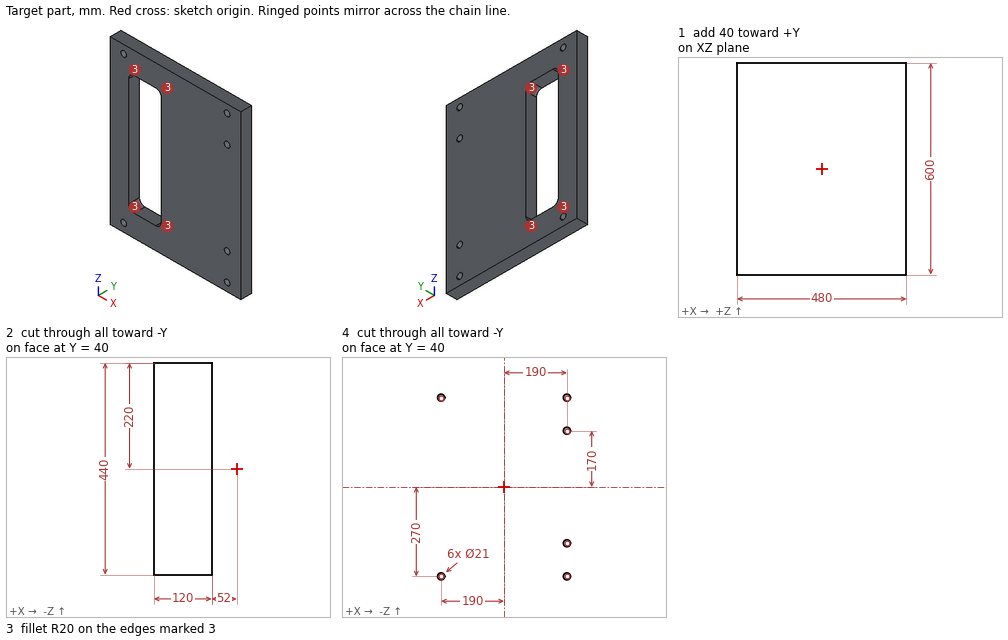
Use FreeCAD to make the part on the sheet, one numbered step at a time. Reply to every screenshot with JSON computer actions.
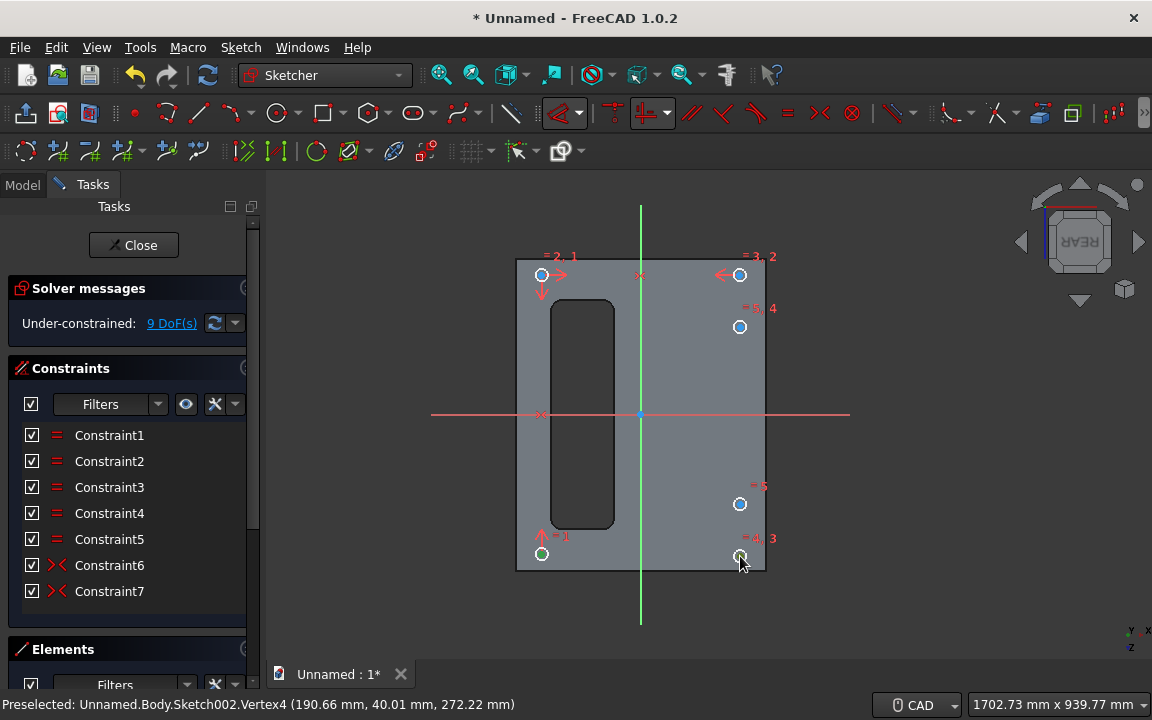
{"action": "left_click", "coordinate": [641, 600]}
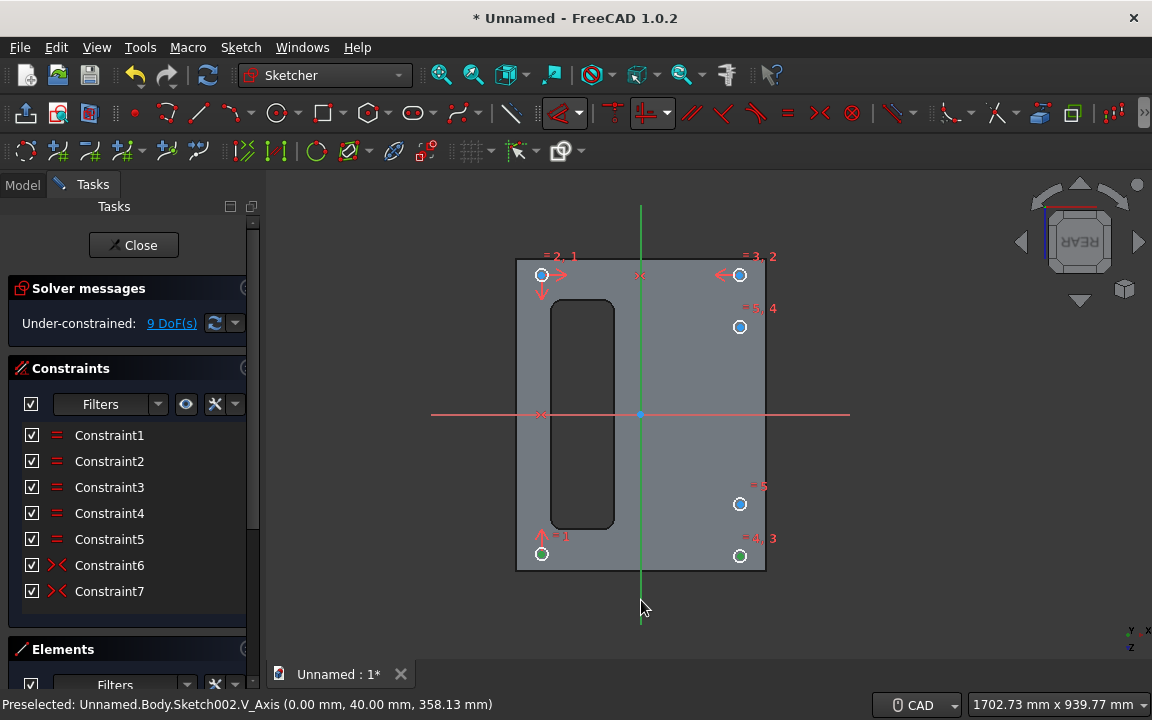
{"action": "left_click", "coordinate": [820, 114]}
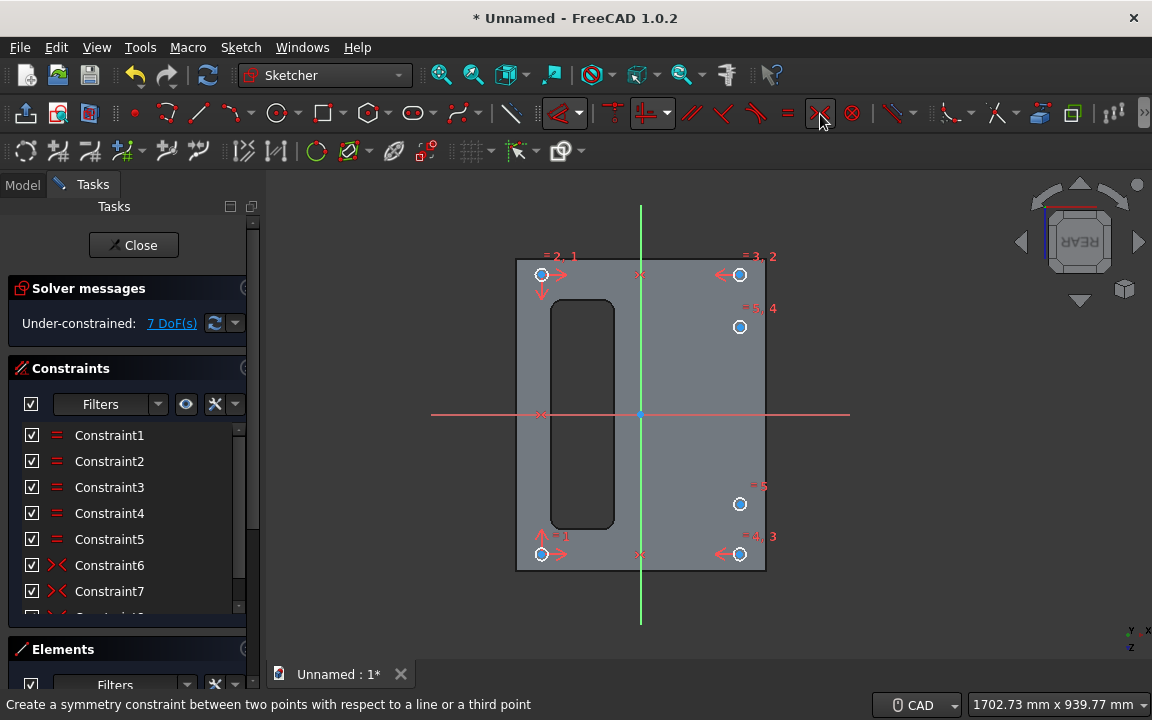
{"action": "left_click", "coordinate": [740, 327]}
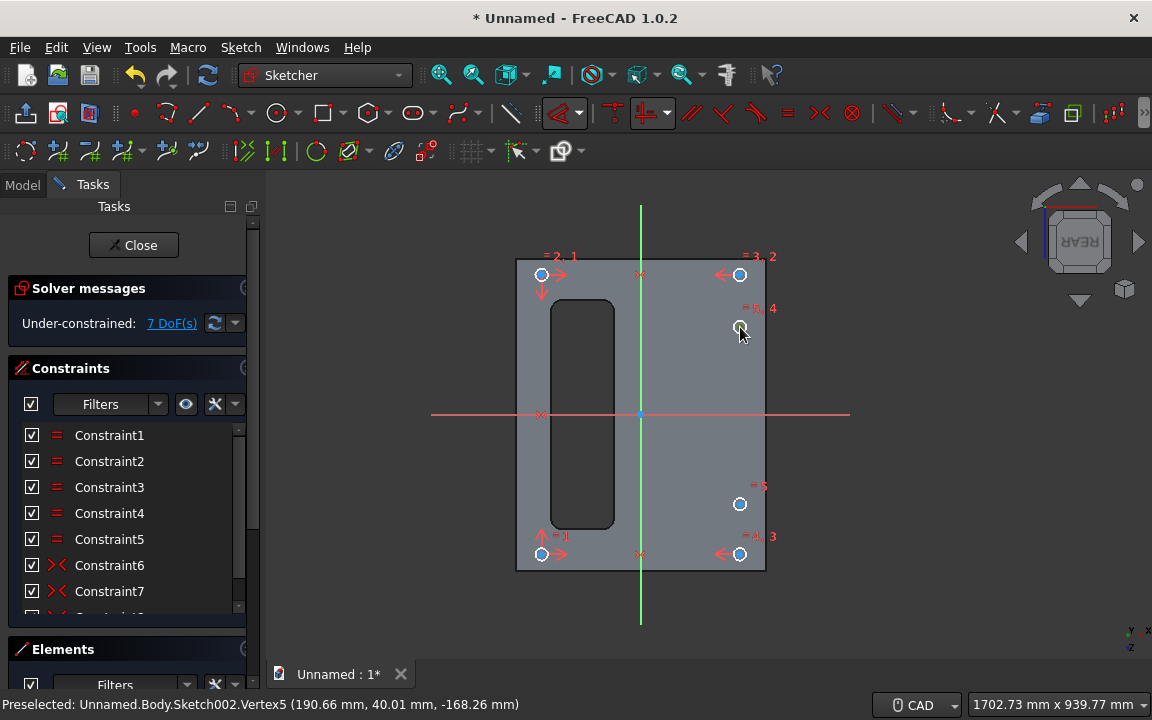
{"action": "left_click", "coordinate": [740, 504]}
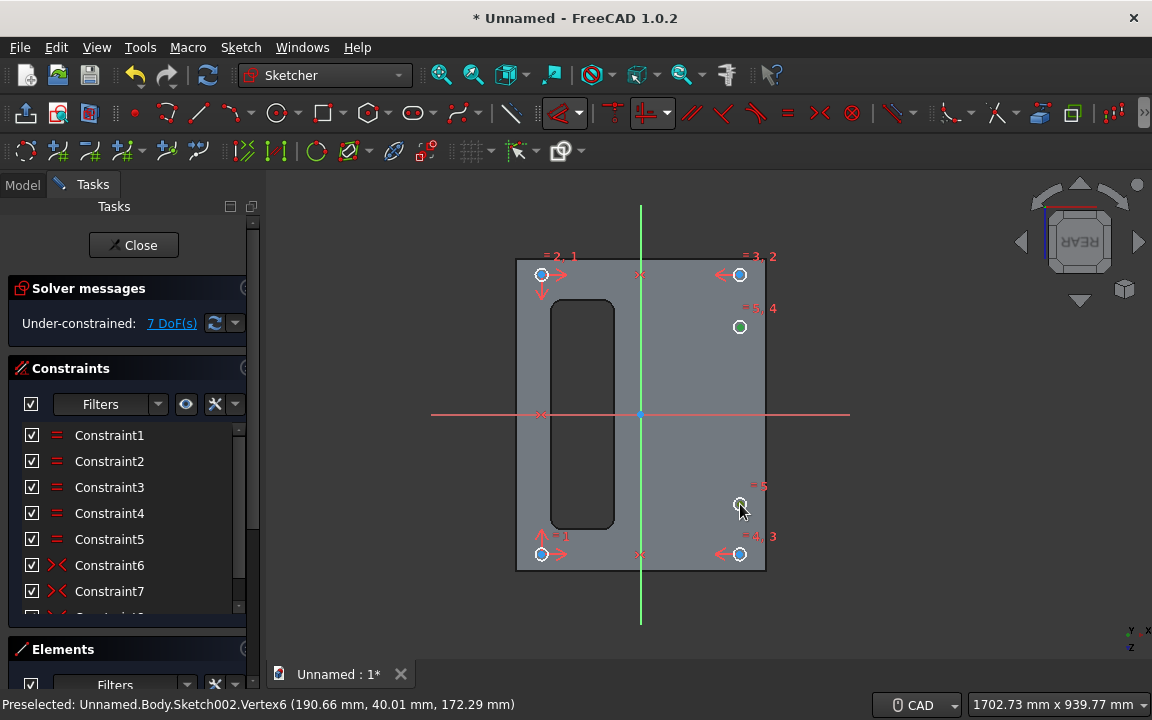
{"action": "left_click", "coordinate": [442, 415]}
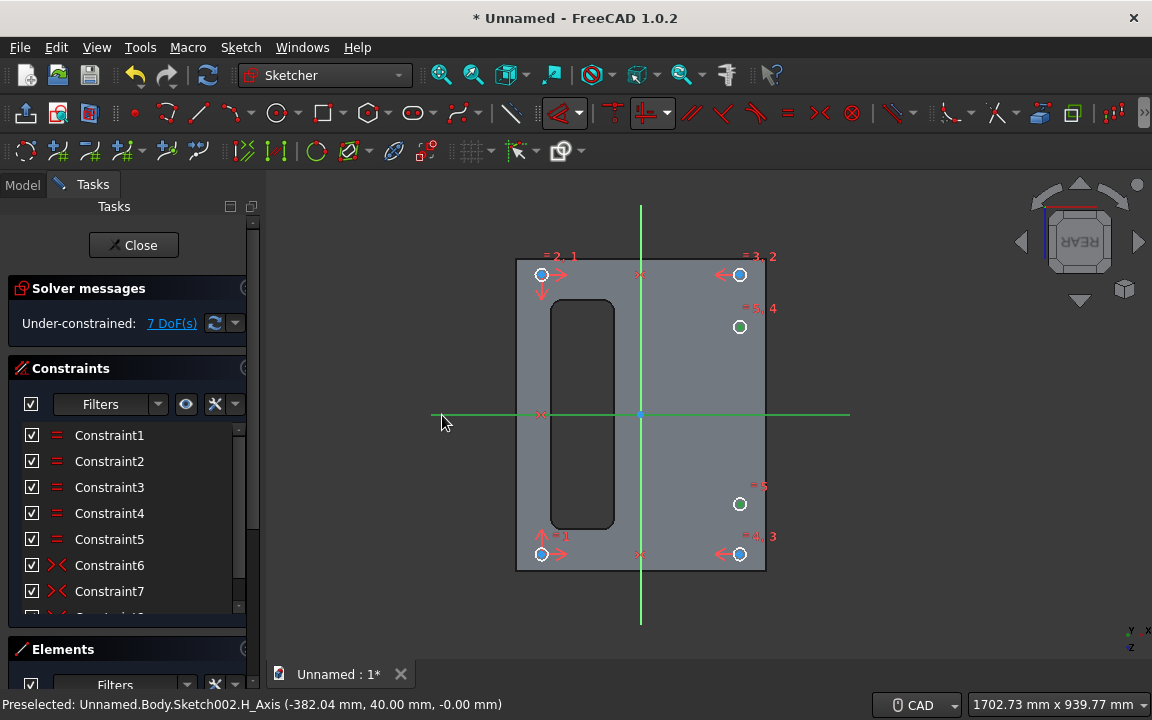
{"action": "key", "text": "s"}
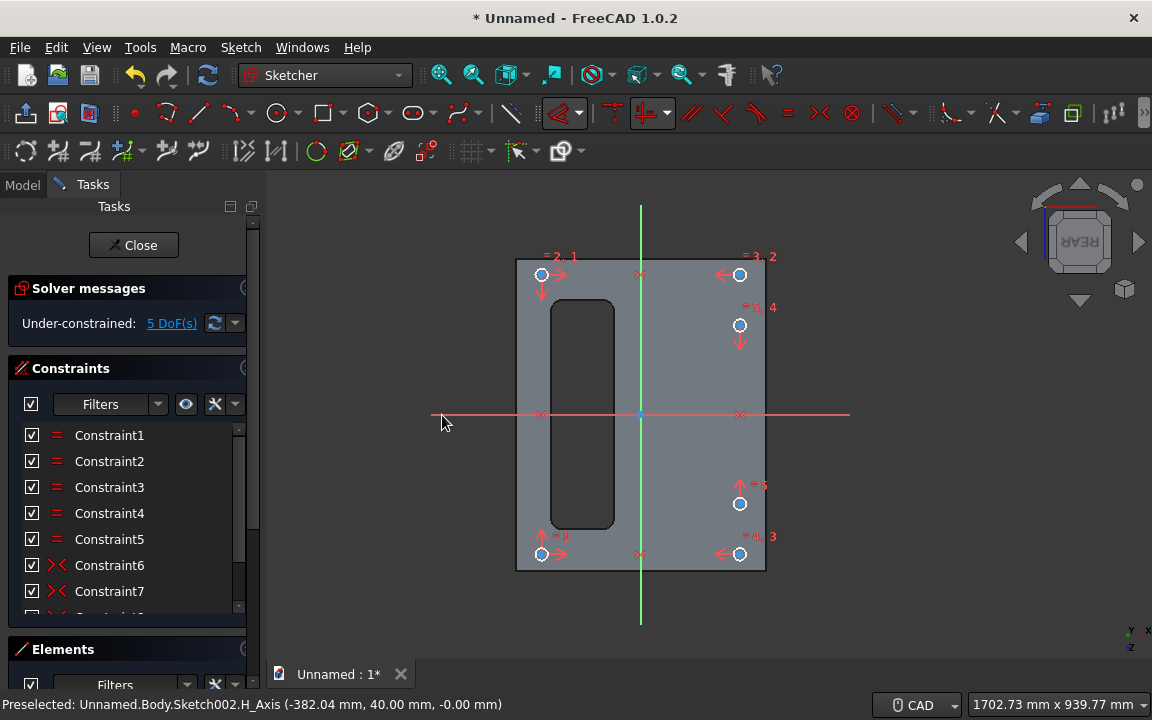
{"action": "scroll", "coordinate": [537, 559], "scroll_direction": "up", "scroll_amount": 7}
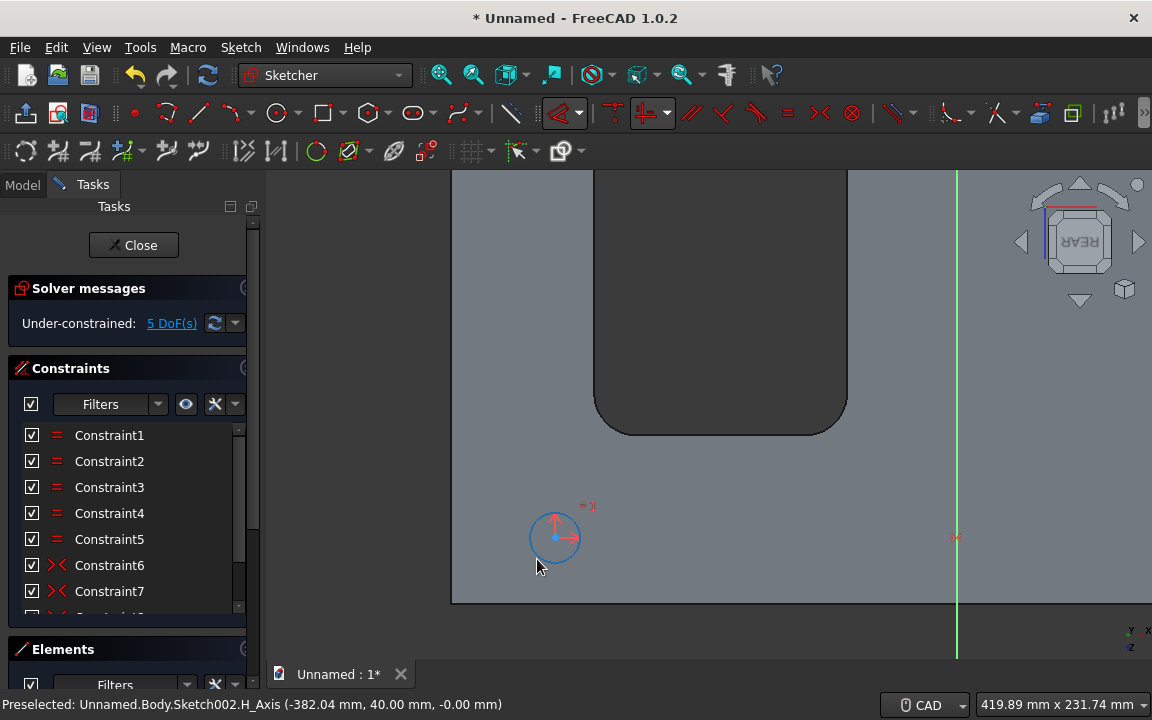
{"action": "left_click", "coordinate": [537, 556]}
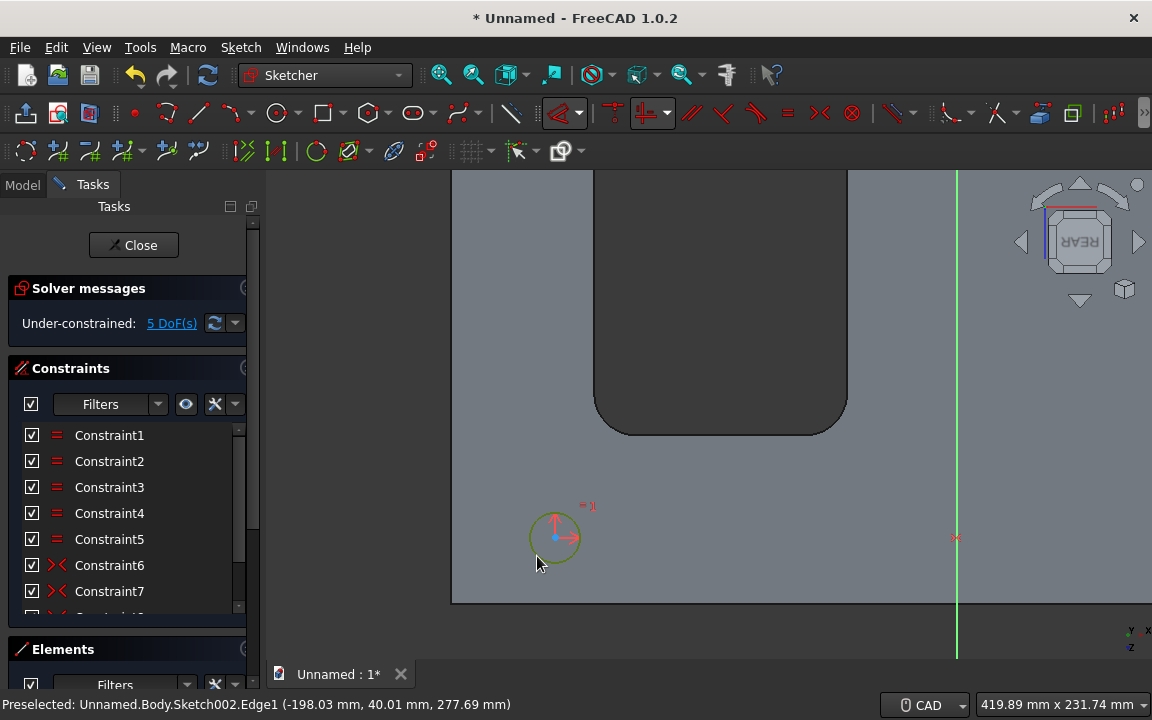
{"action": "key", "text": "k o"}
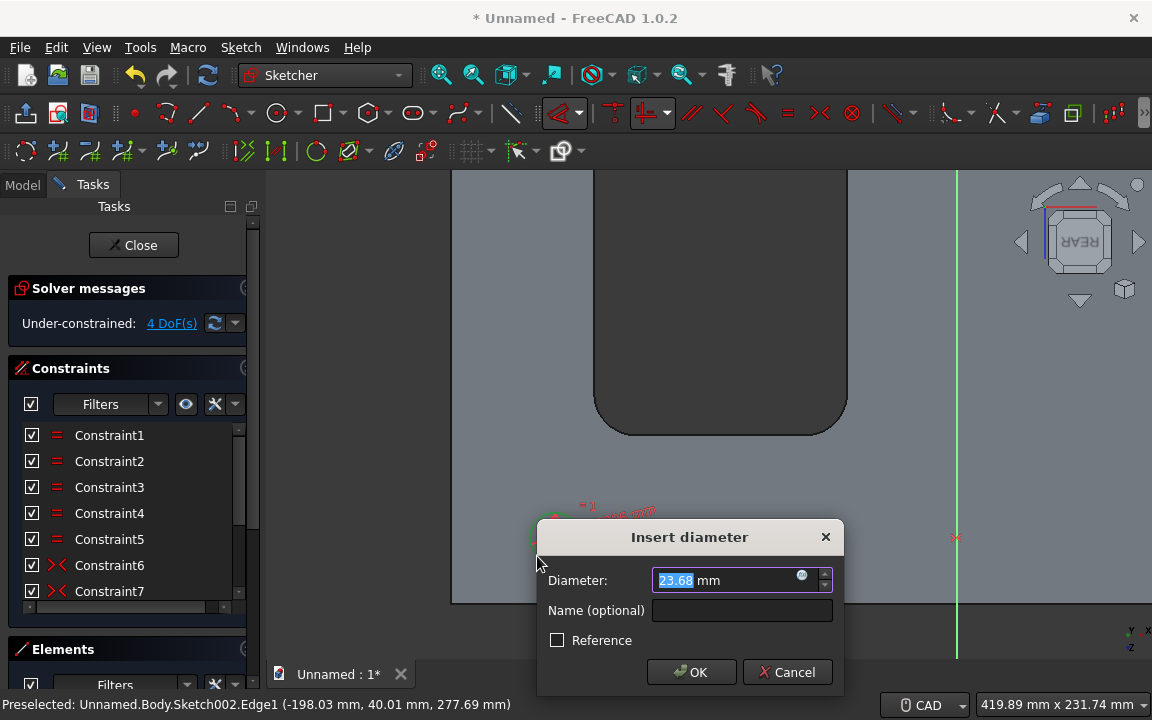
{"action": "type", "text": "21"}
{"action": "key", "text": "Return"}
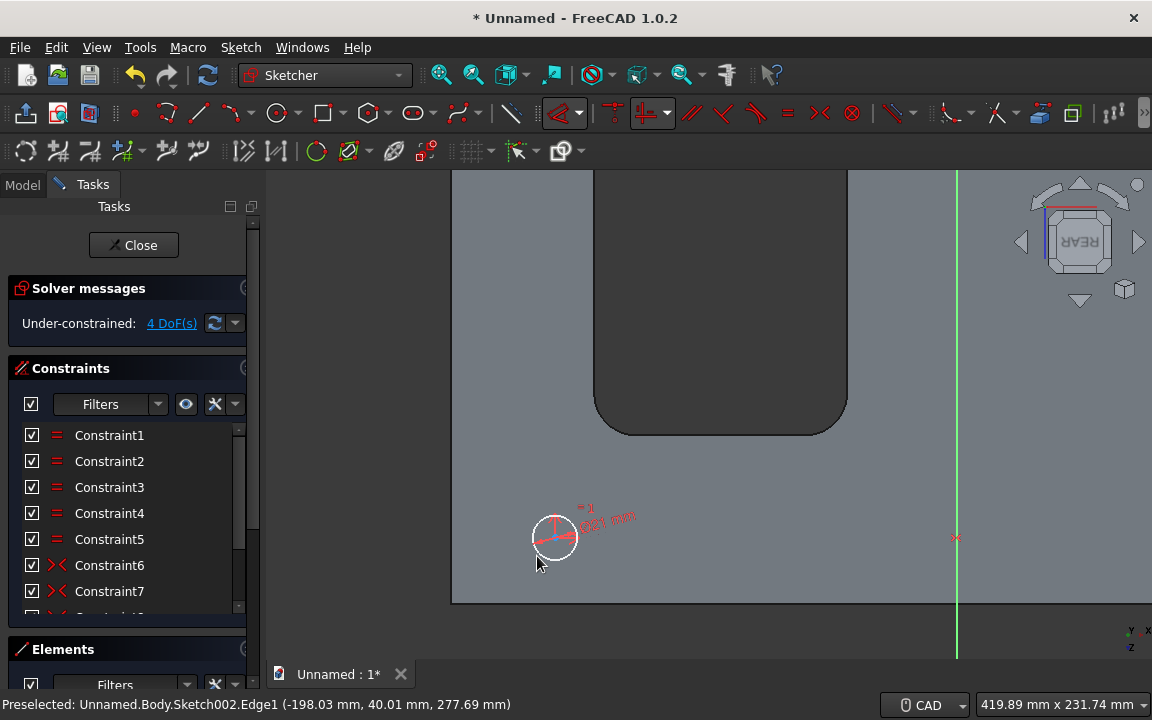
{"action": "left_click", "coordinate": [555, 538]}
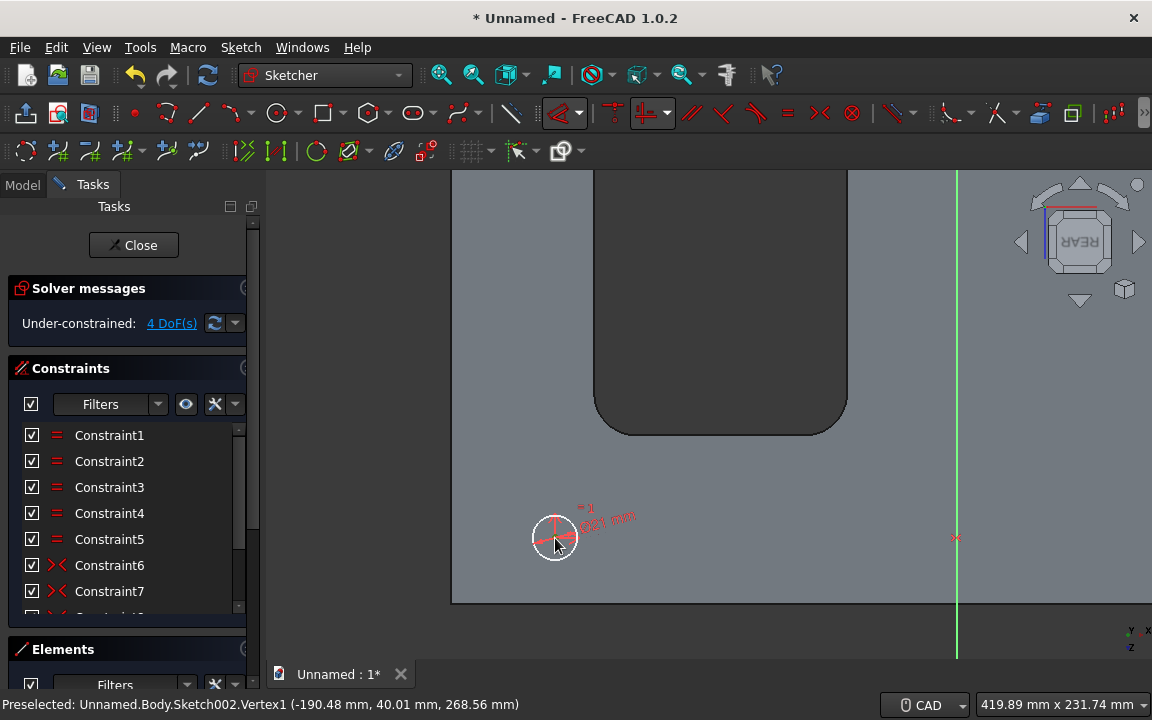
{"action": "left_click", "coordinate": [582, 114]}